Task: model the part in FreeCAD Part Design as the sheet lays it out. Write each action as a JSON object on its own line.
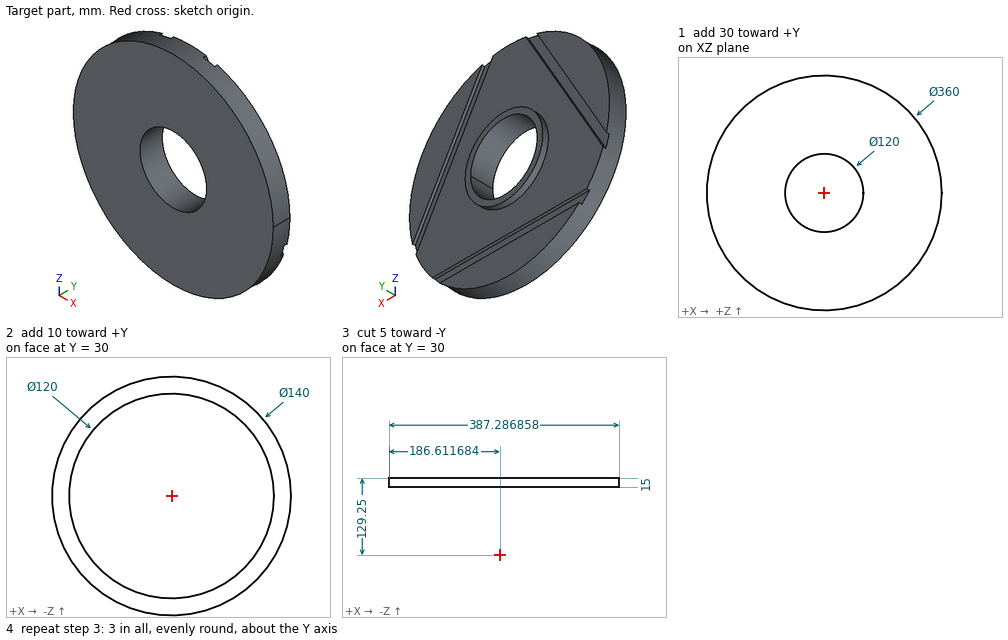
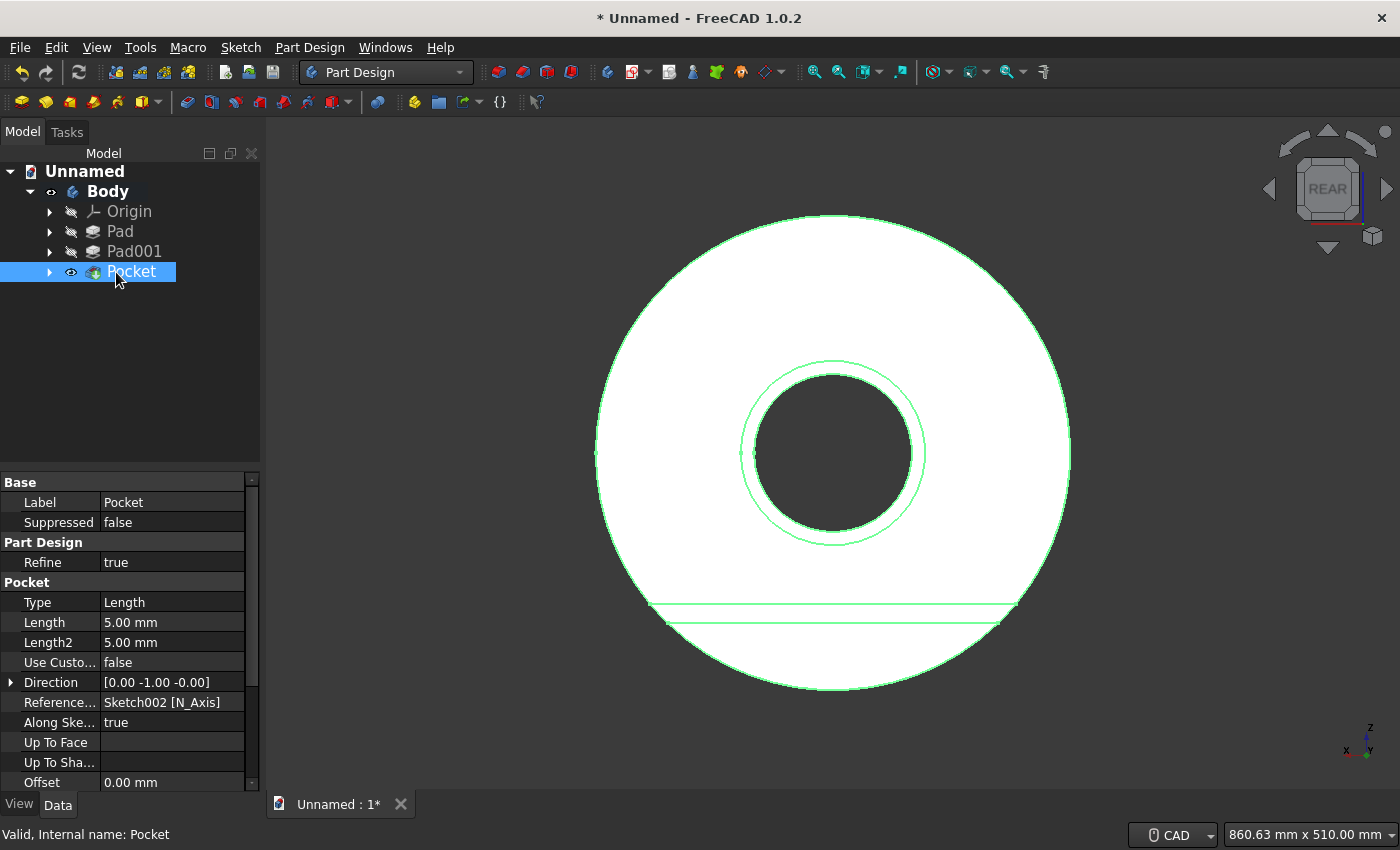
{"action": "left_click", "coordinate": [164, 72]}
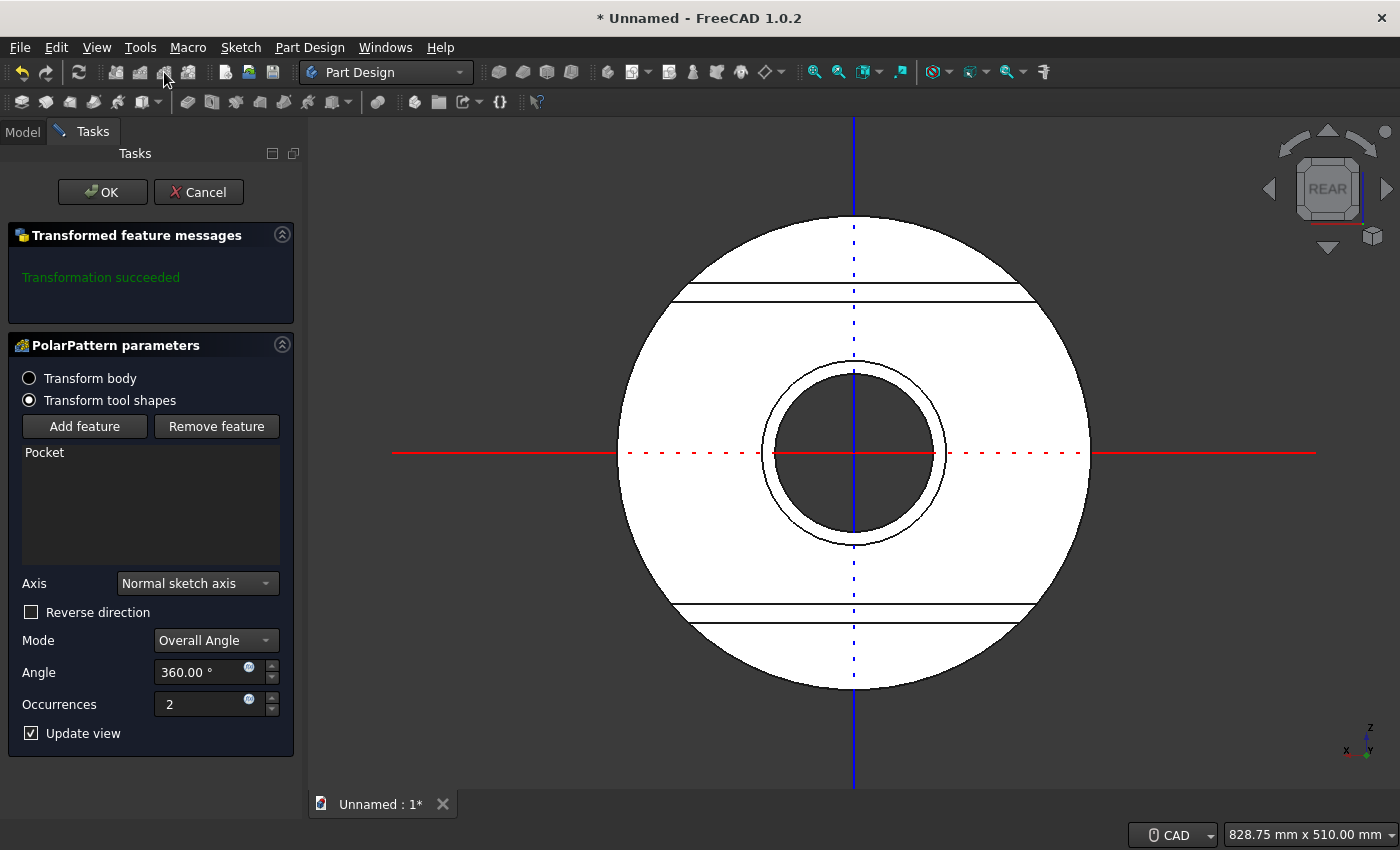
{"action": "left_click", "coordinate": [198, 584]}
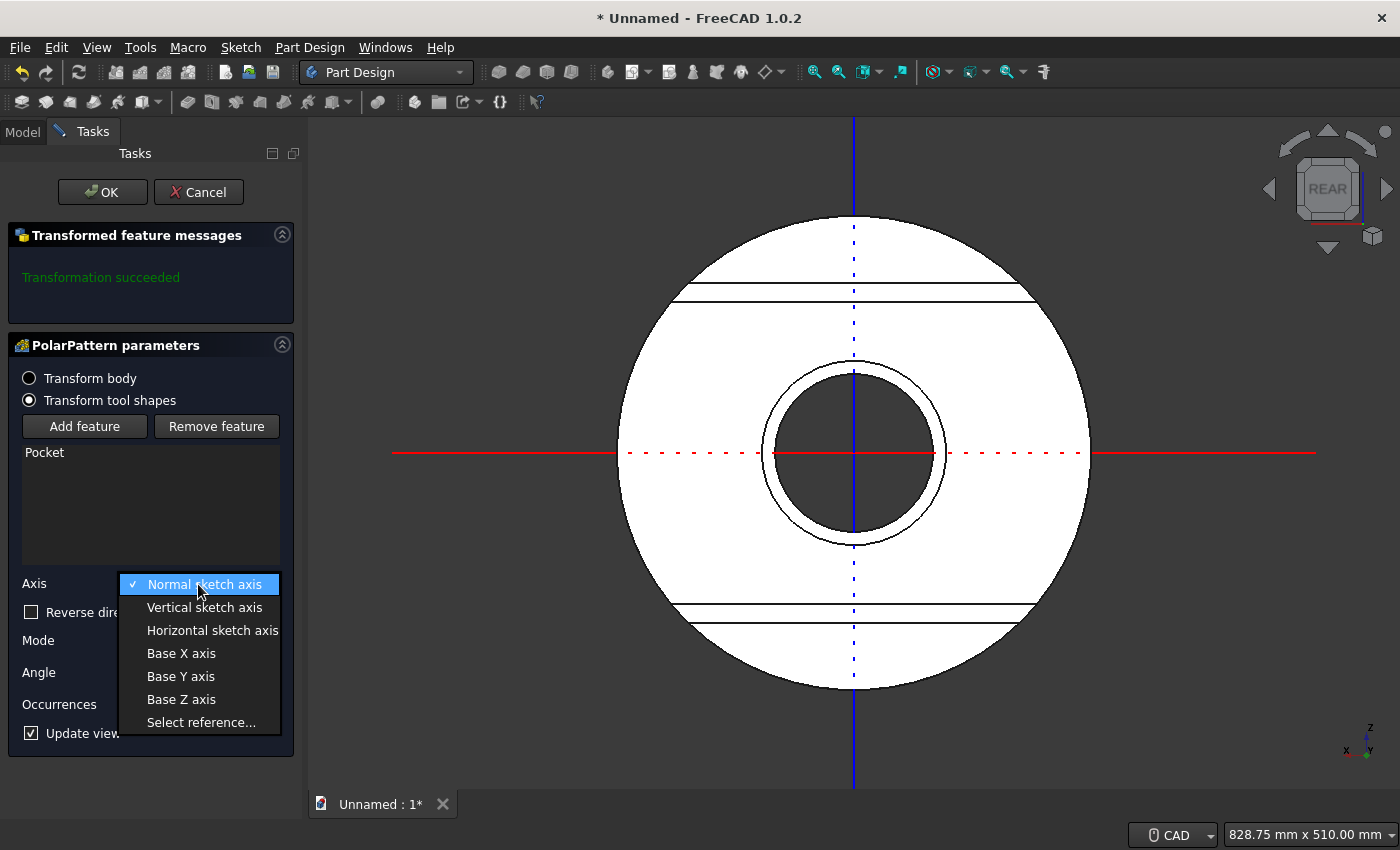
{"action": "left_click", "coordinate": [198, 676]}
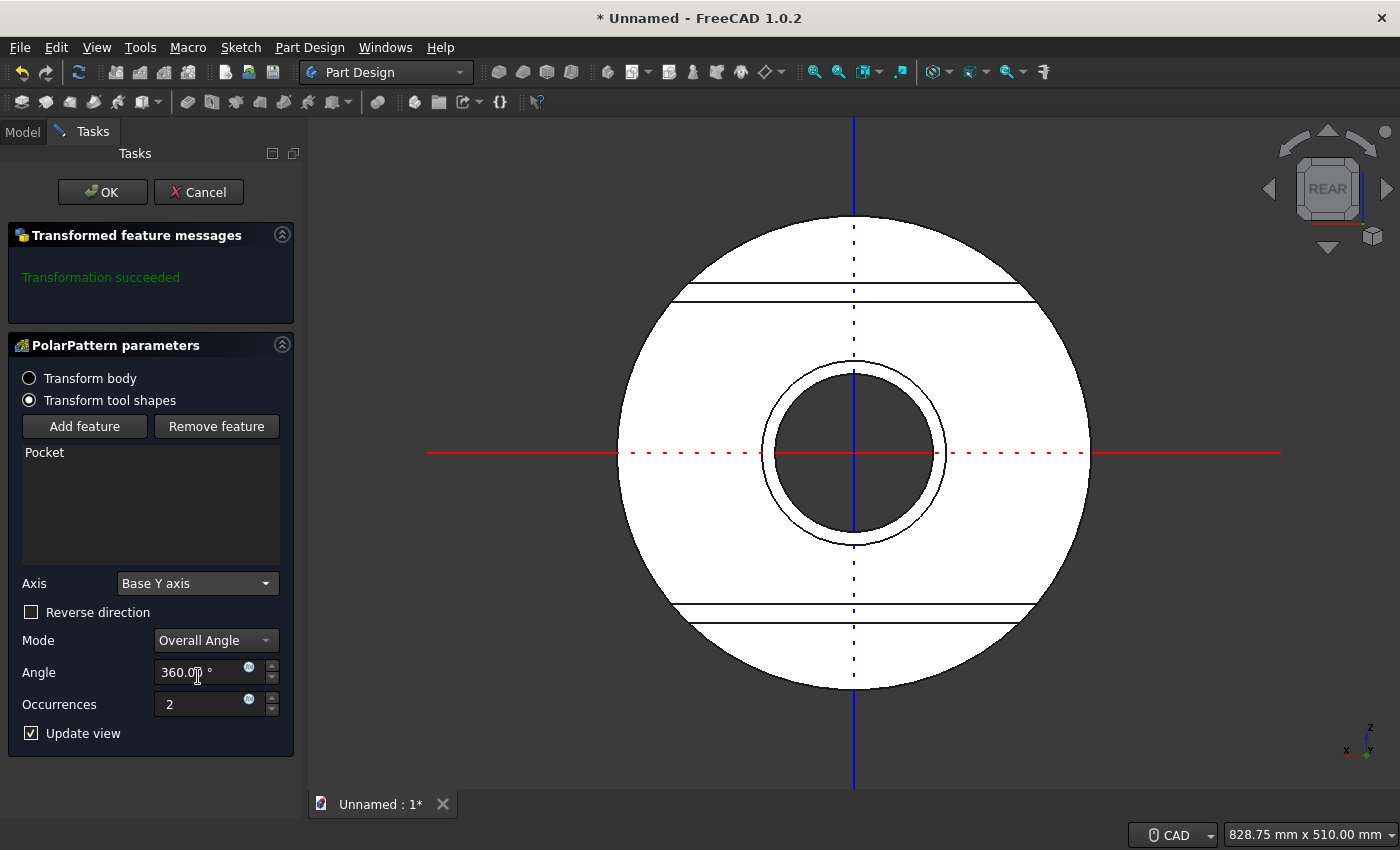
{"action": "triple_click", "coordinate": [209, 704]}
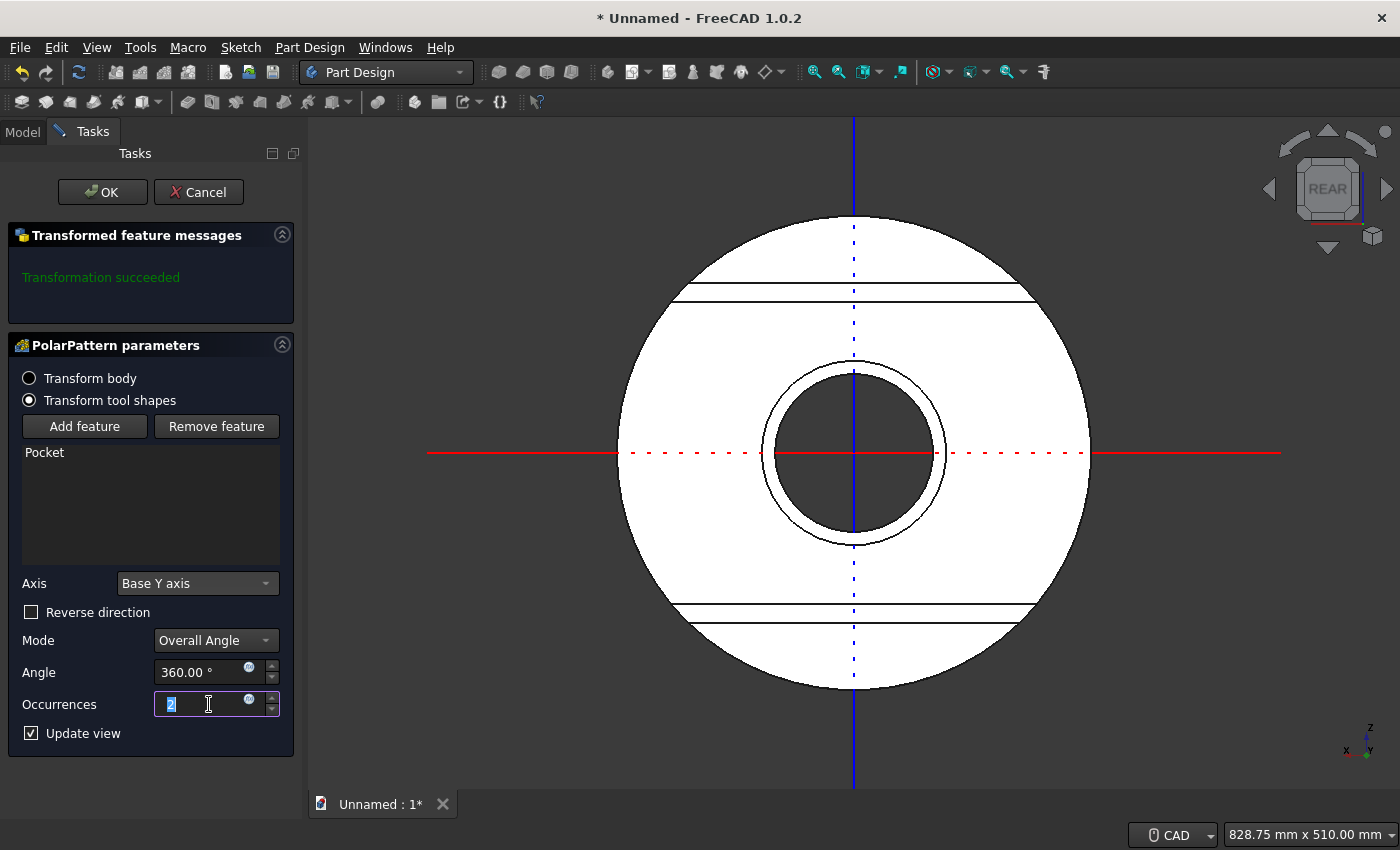
{"action": "type", "text": "3"}
{"action": "key", "text": "Tab"}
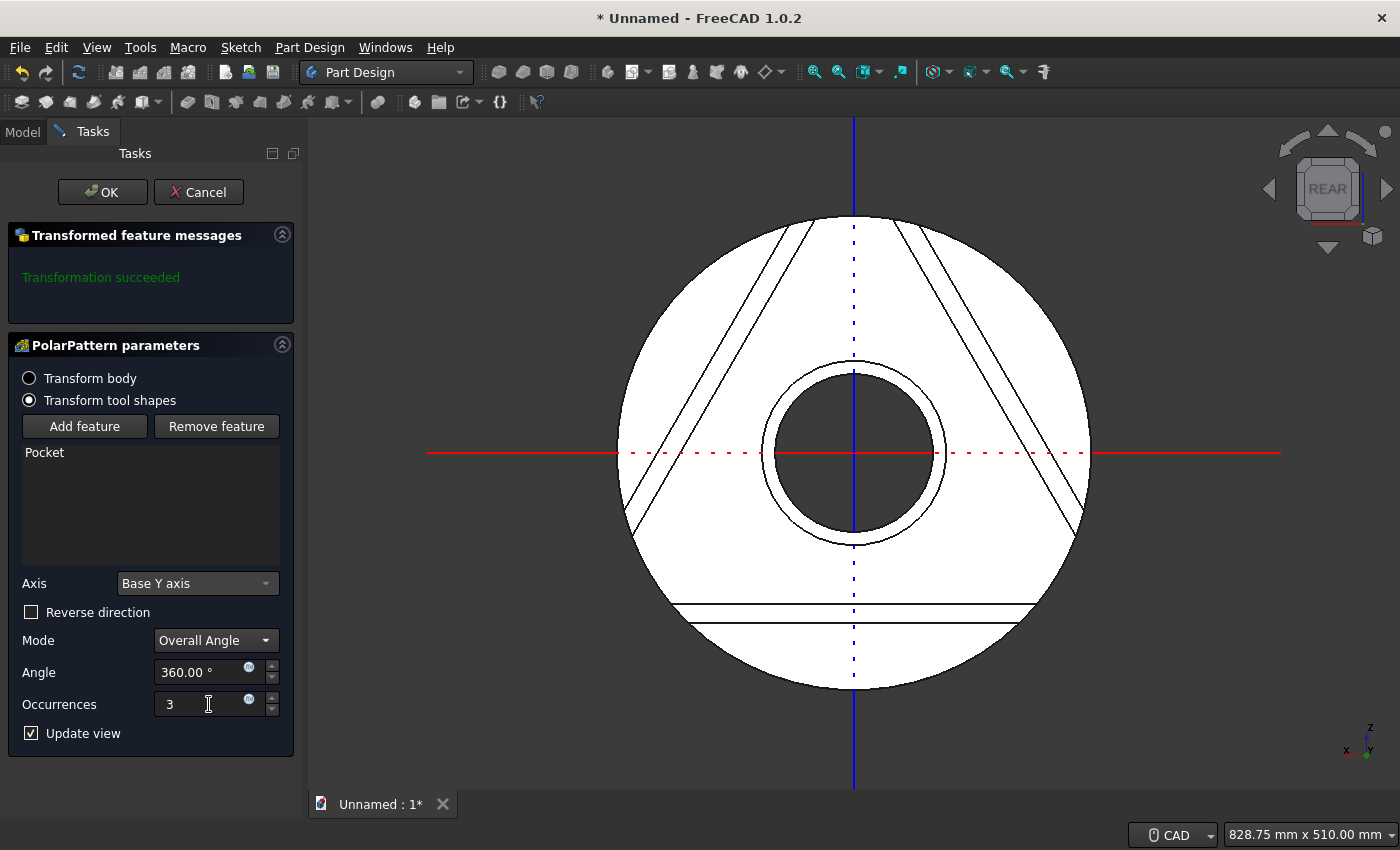
{"action": "left_click", "coordinate": [103, 192]}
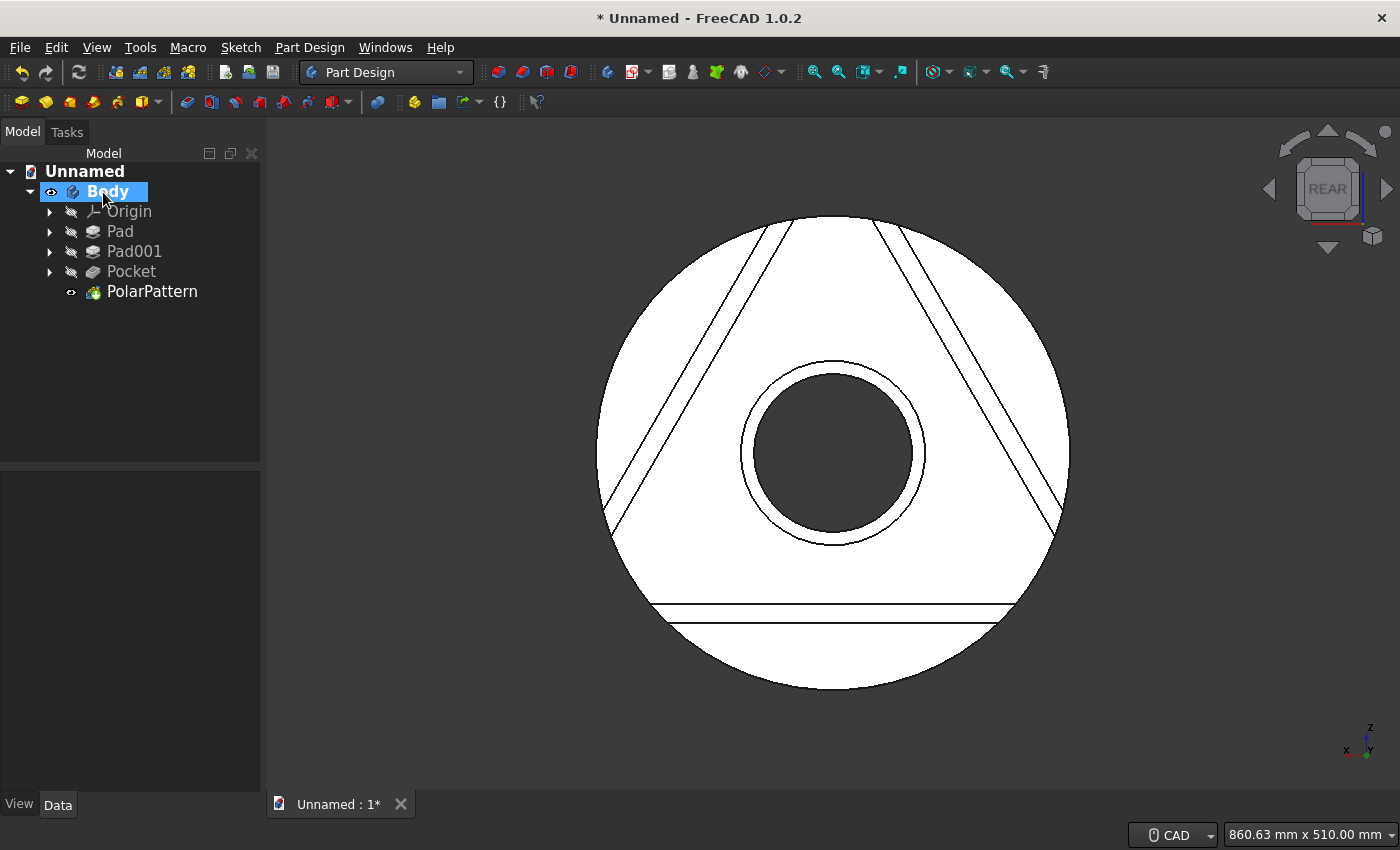
{"action": "key", "text": "0"}